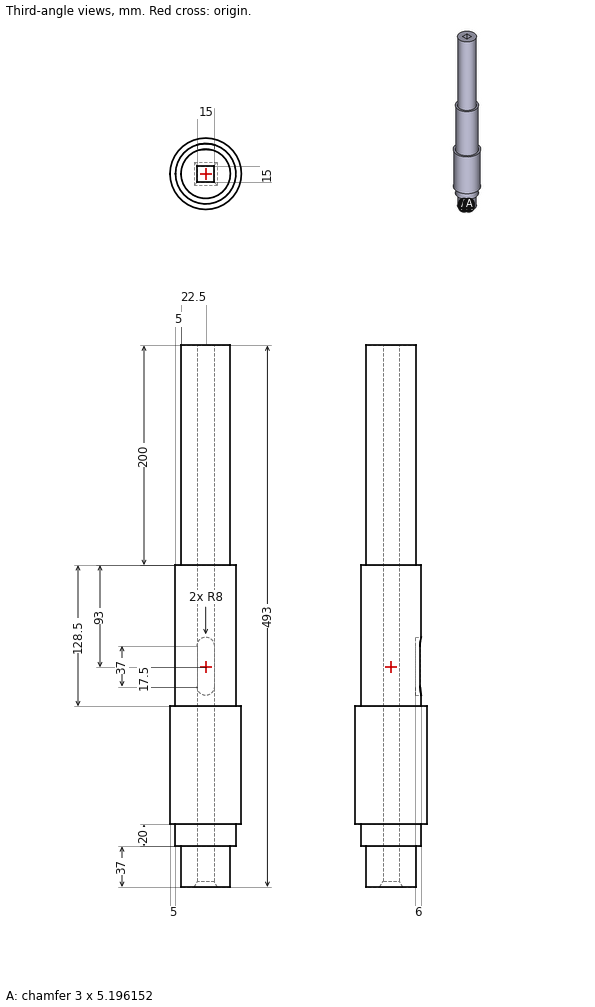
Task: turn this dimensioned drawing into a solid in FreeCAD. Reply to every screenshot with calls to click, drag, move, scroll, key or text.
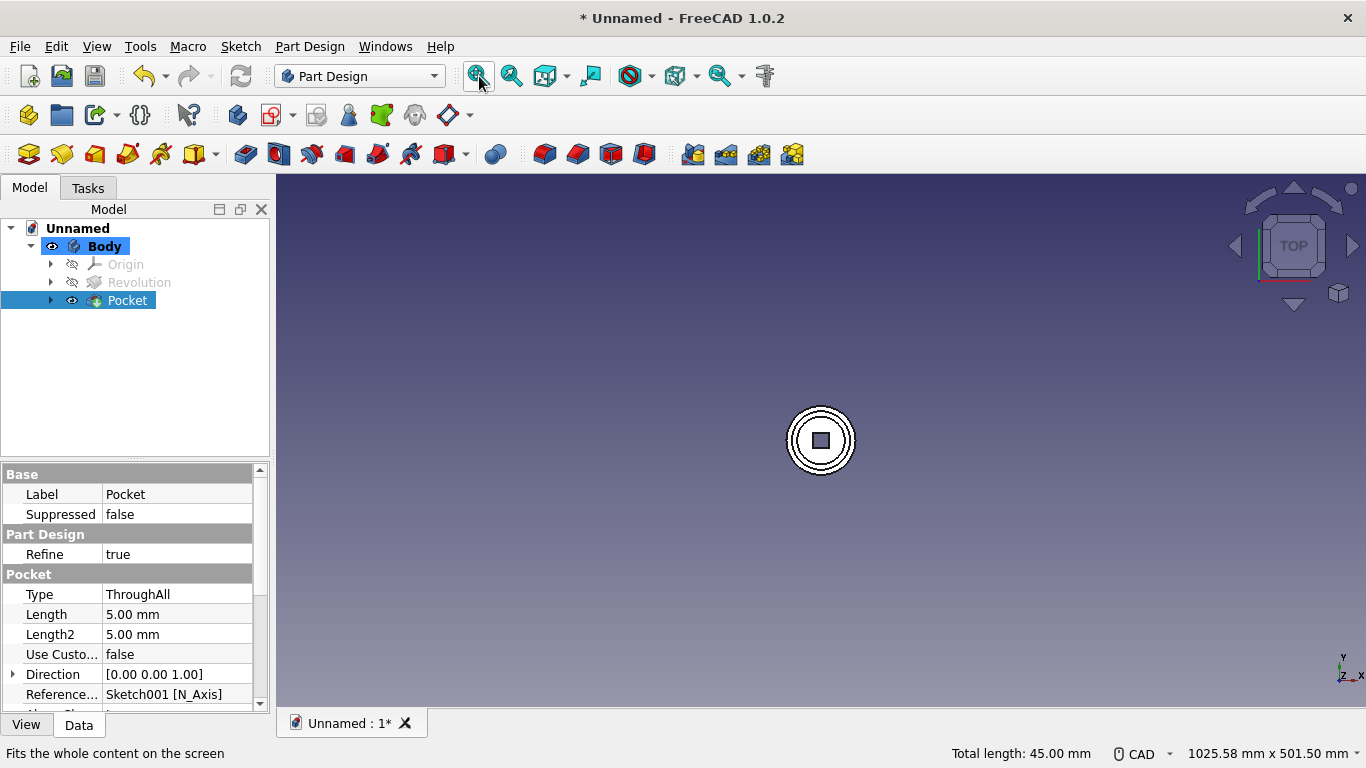
key(v)
key(f)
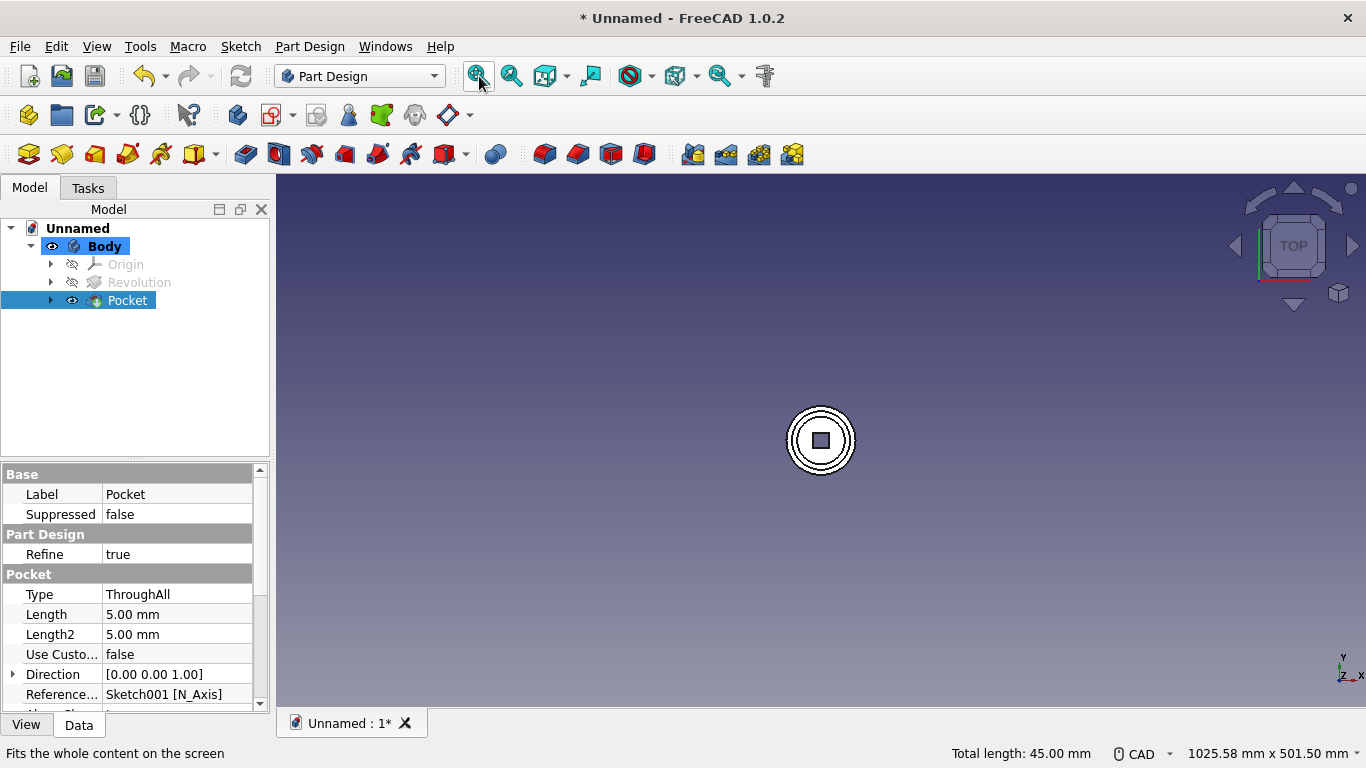
scroll(821, 447, up, 5)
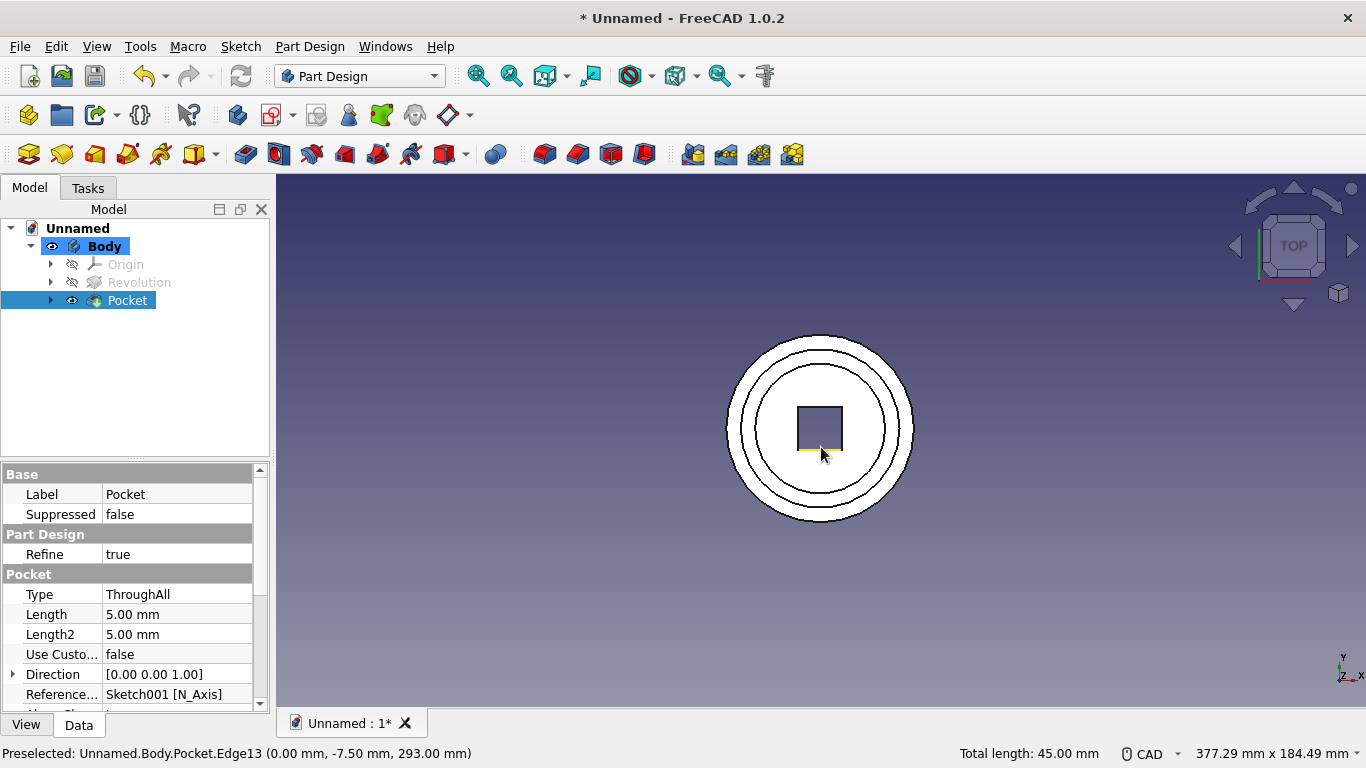
key(v)
key(f)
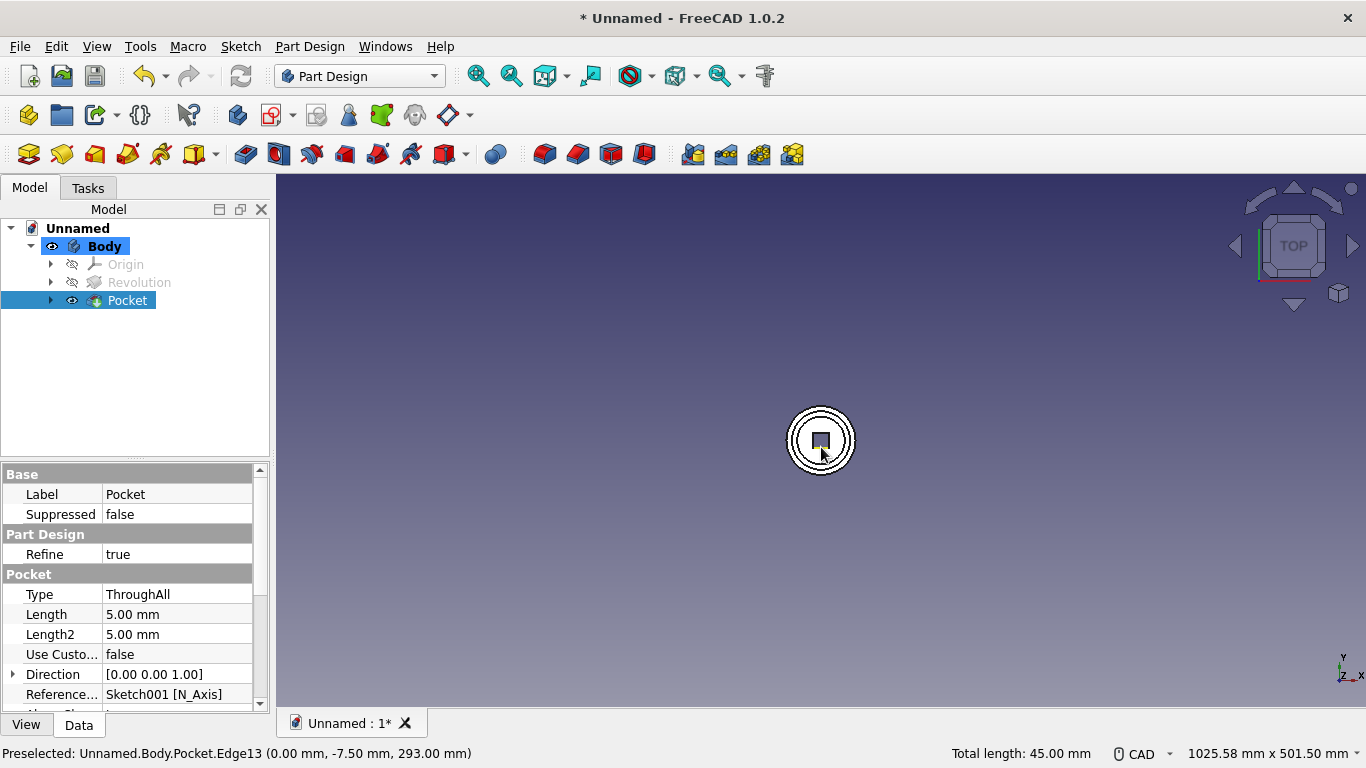
key(1)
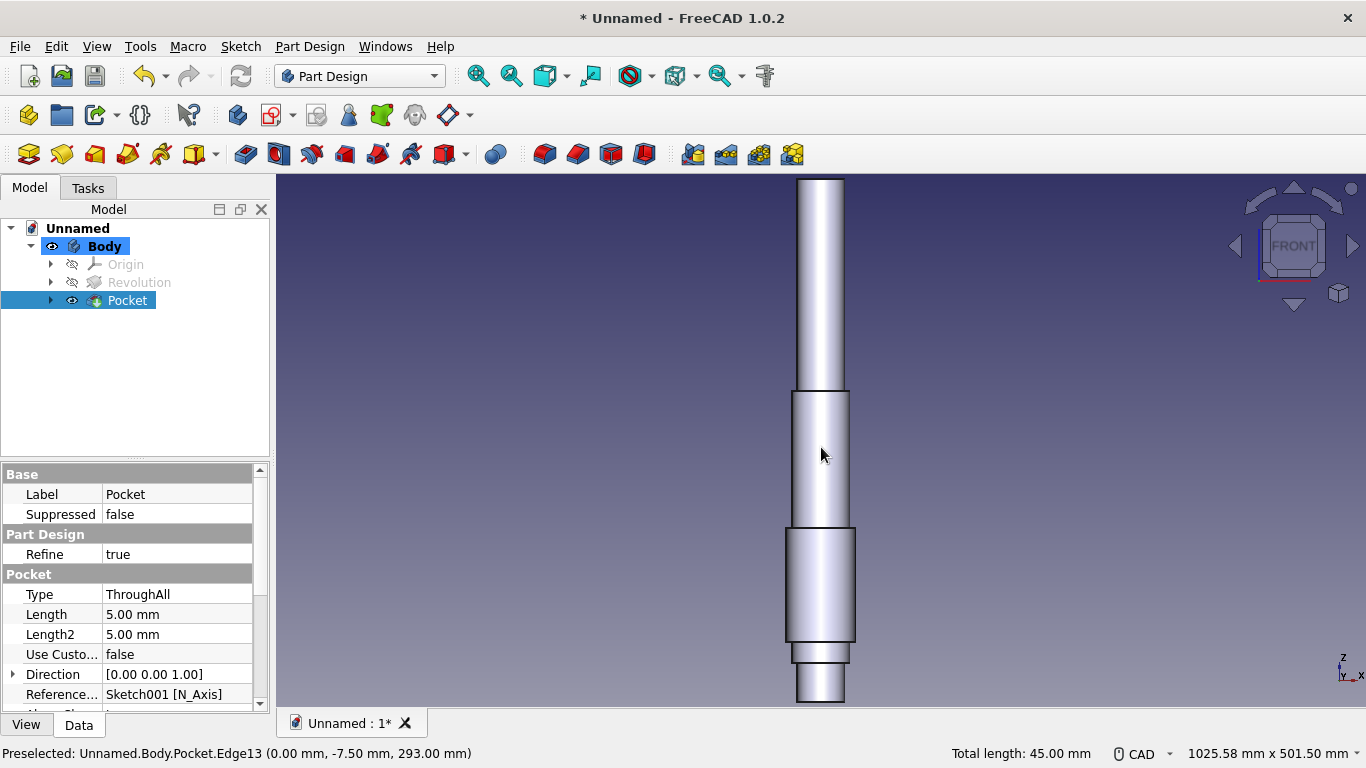
key(3)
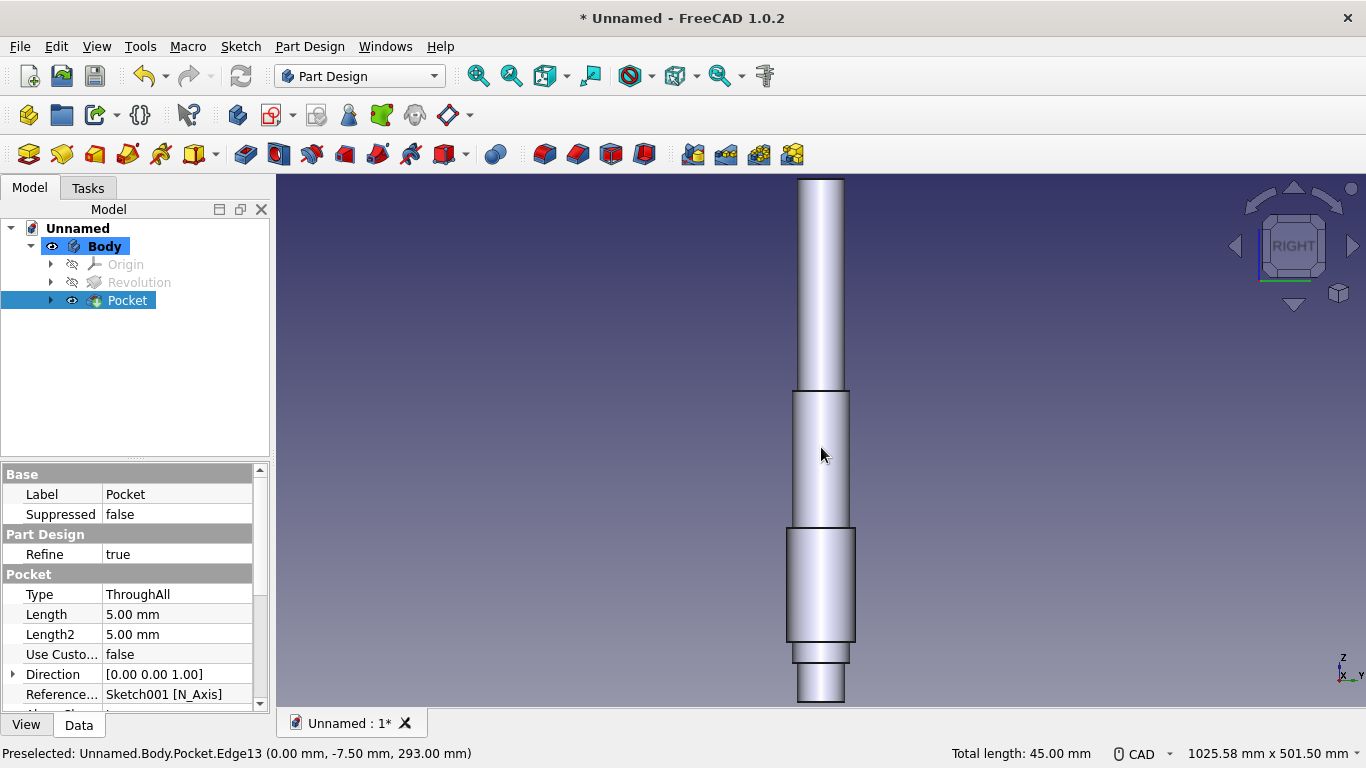
key(5)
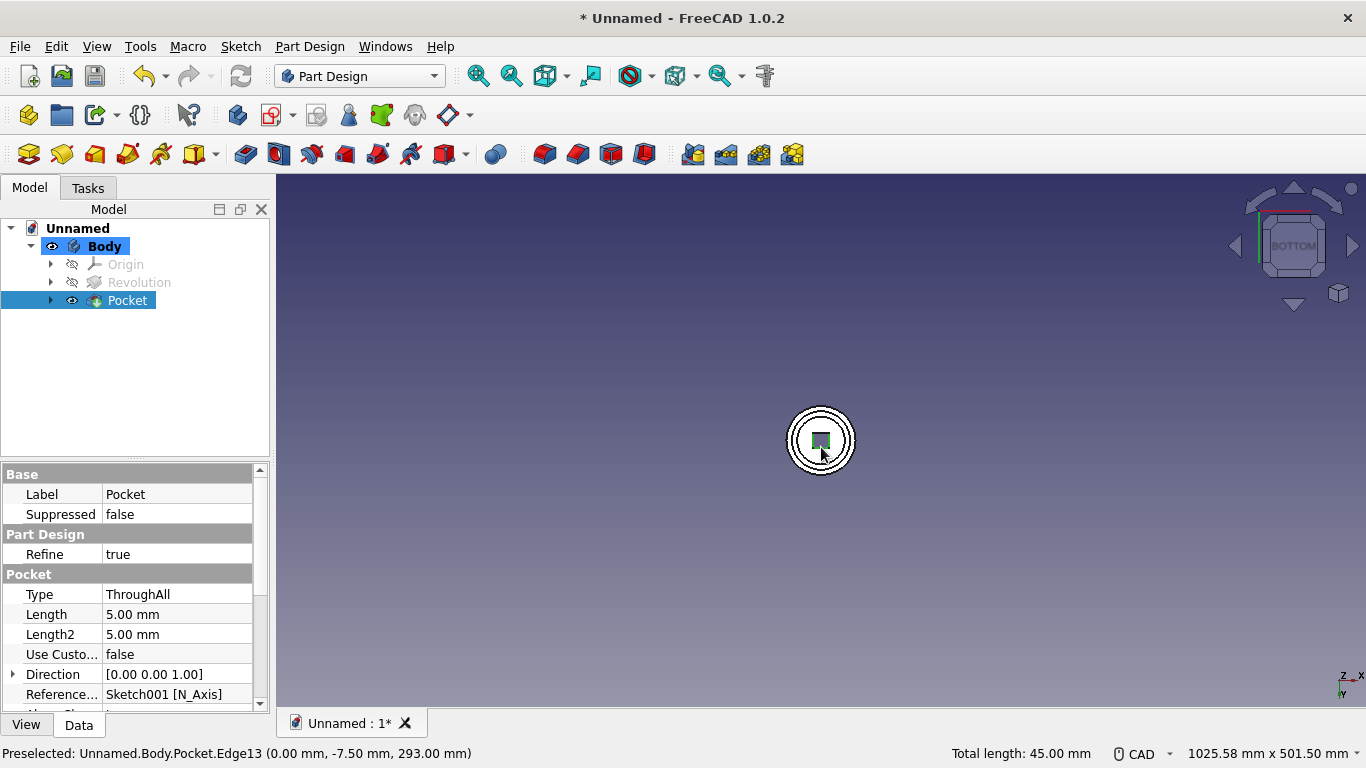
click(479, 76)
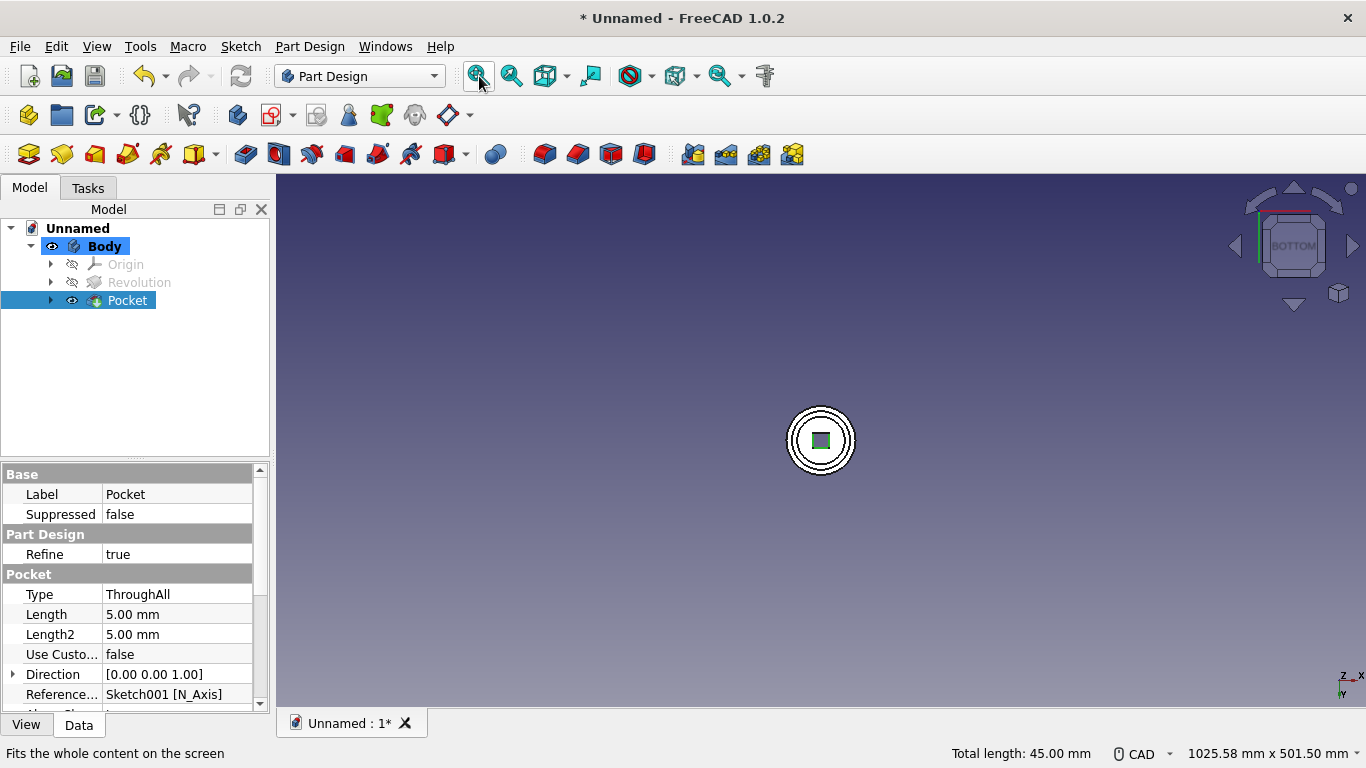
scroll(821, 432, up, 5)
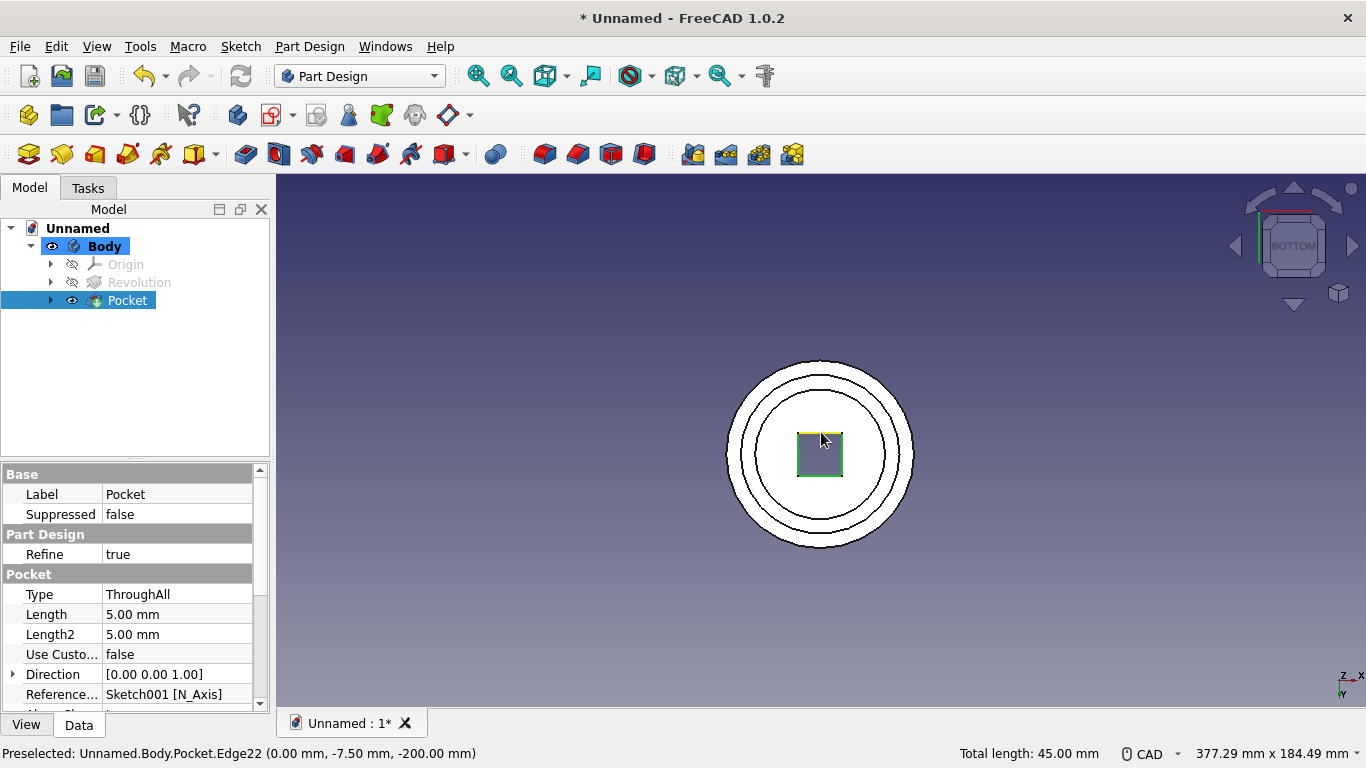
key(v)
key(f)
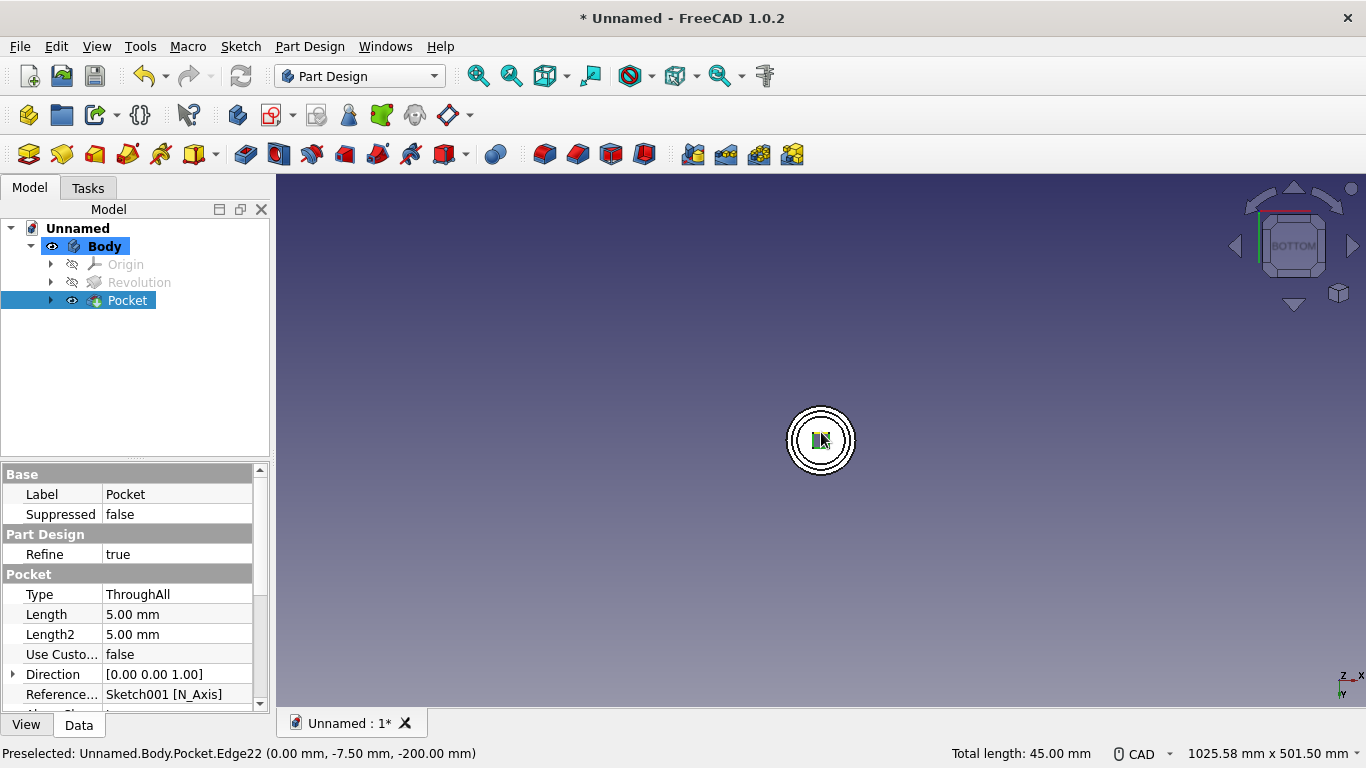
key(4)